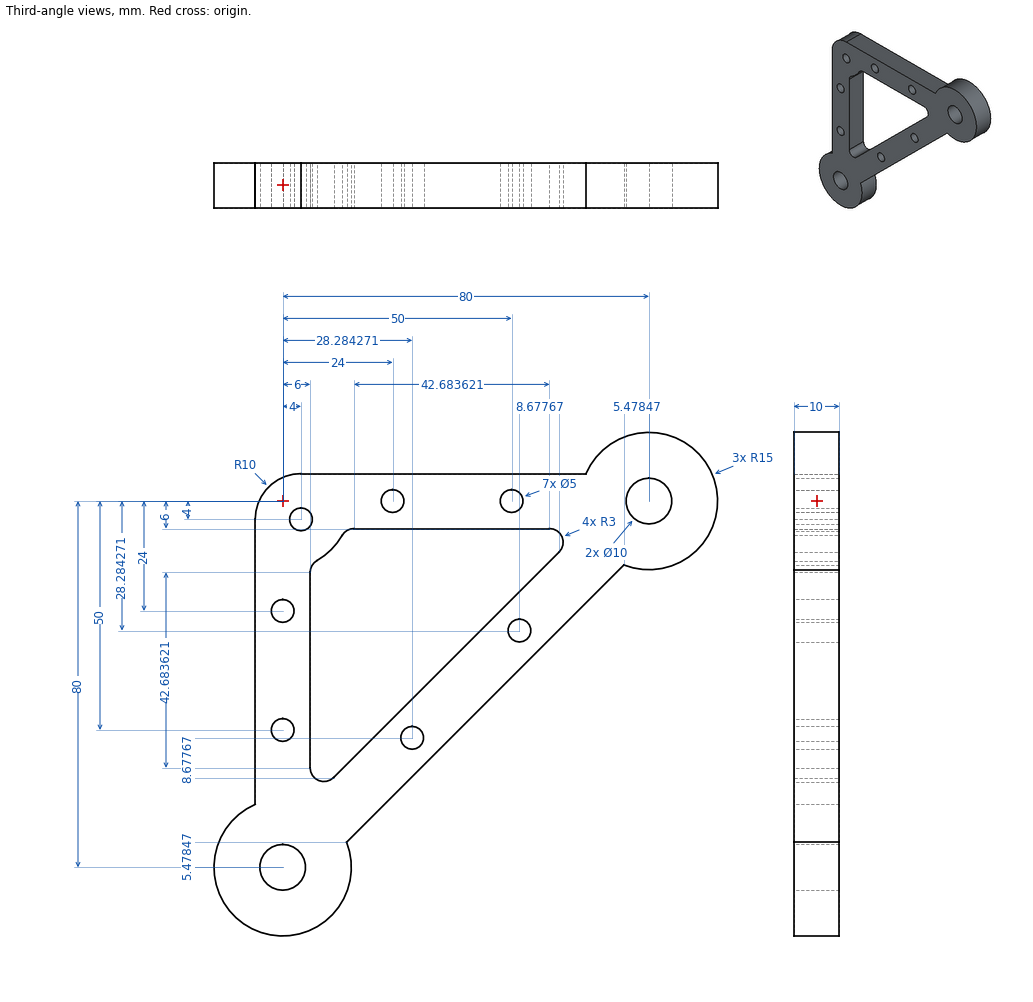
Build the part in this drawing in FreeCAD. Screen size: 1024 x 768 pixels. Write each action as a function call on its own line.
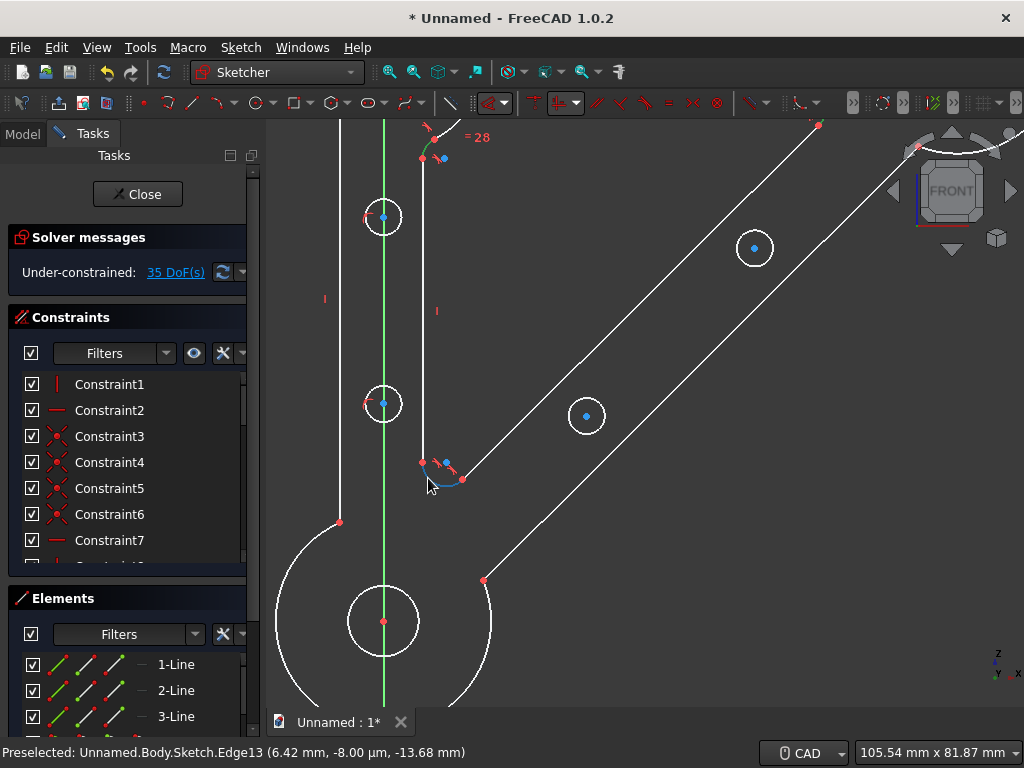
click(428, 478)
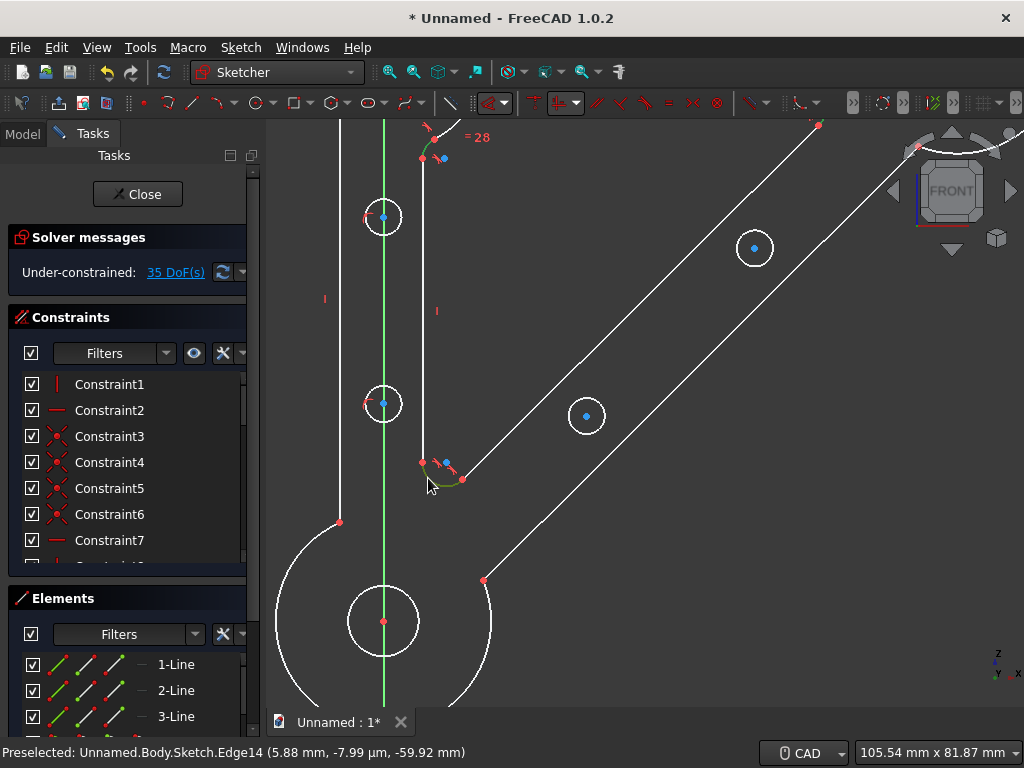
click(670, 104)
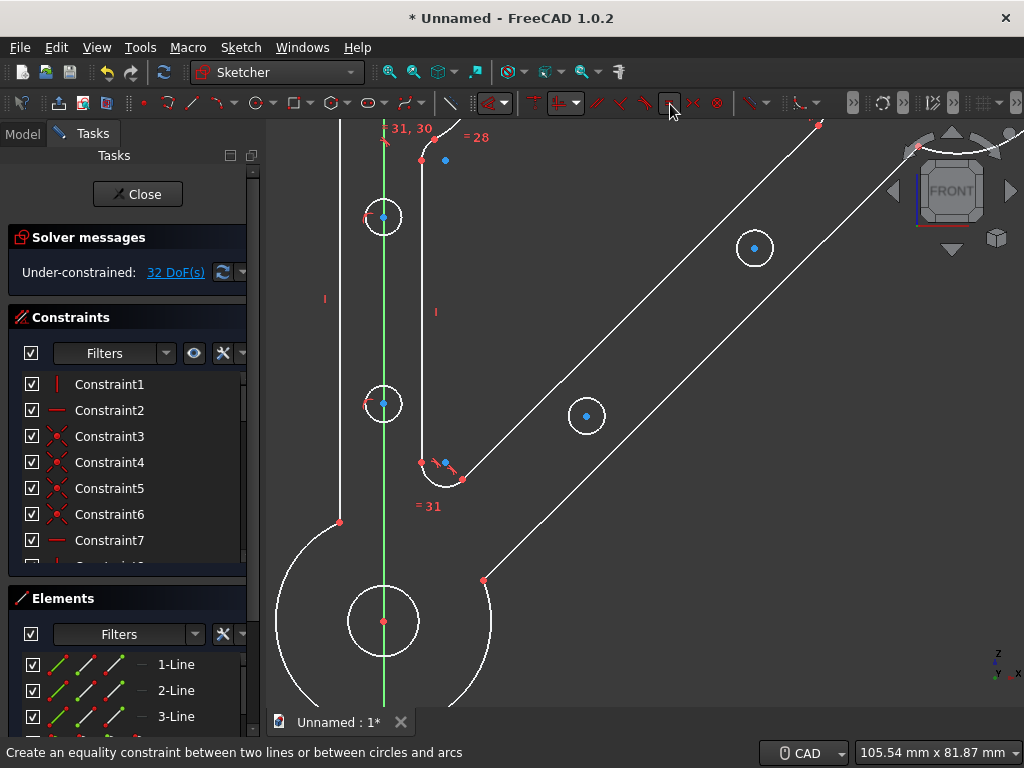
scroll(428, 478, down, 3)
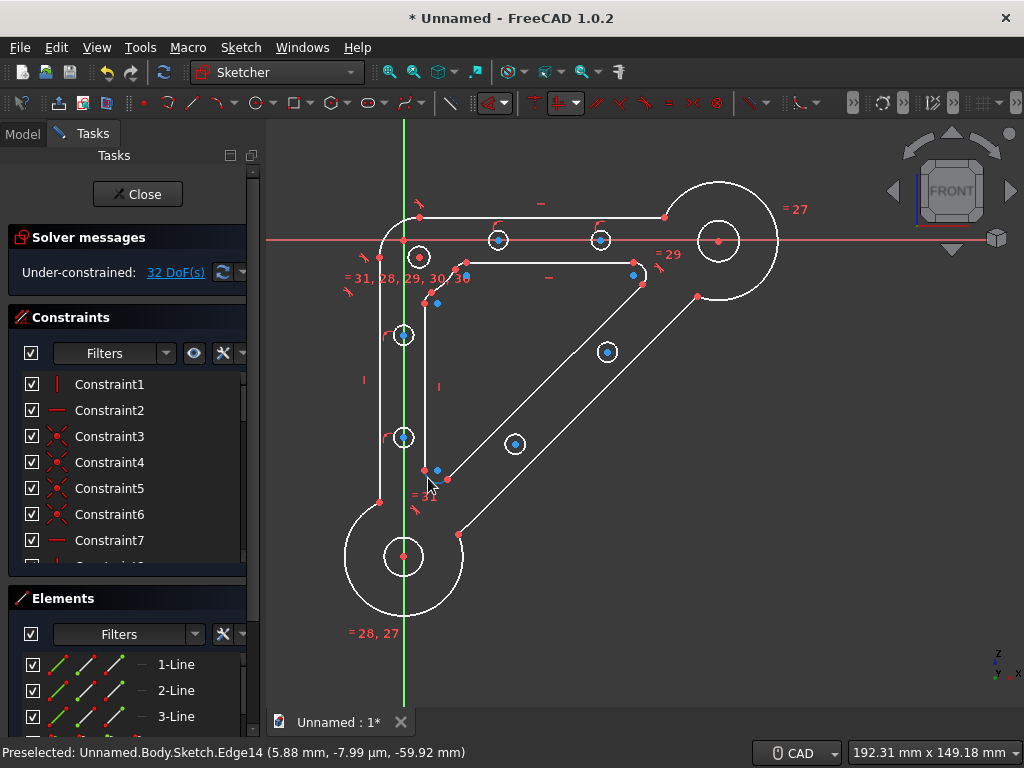
scroll(608, 233, up, 4)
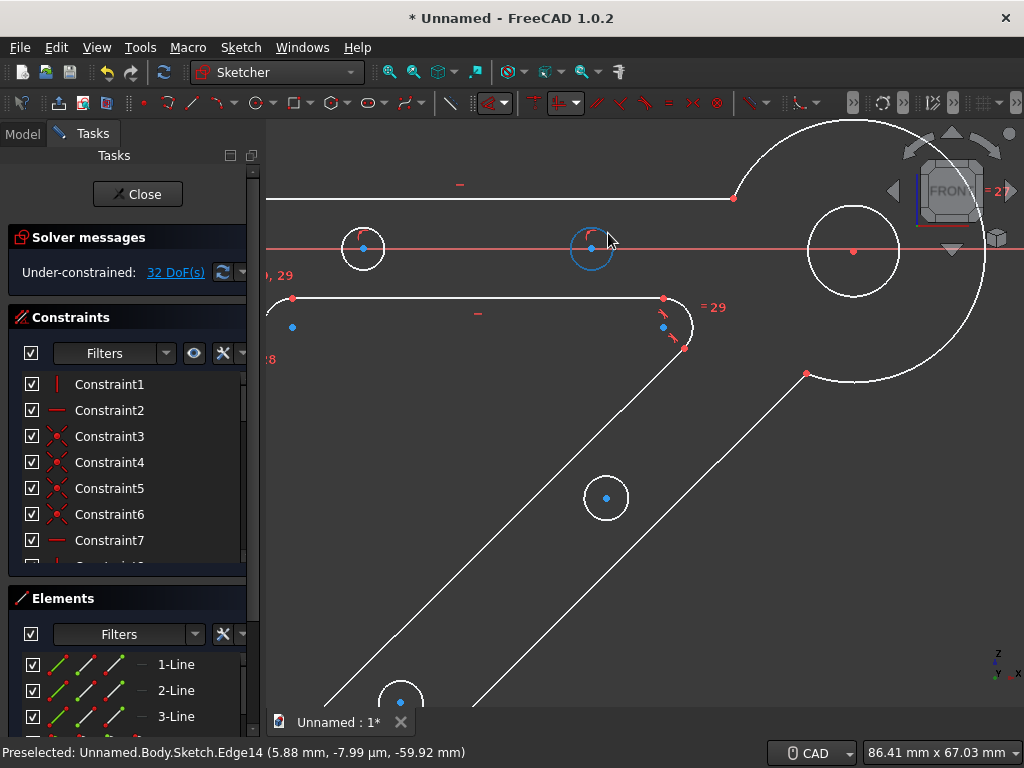
click(607, 234)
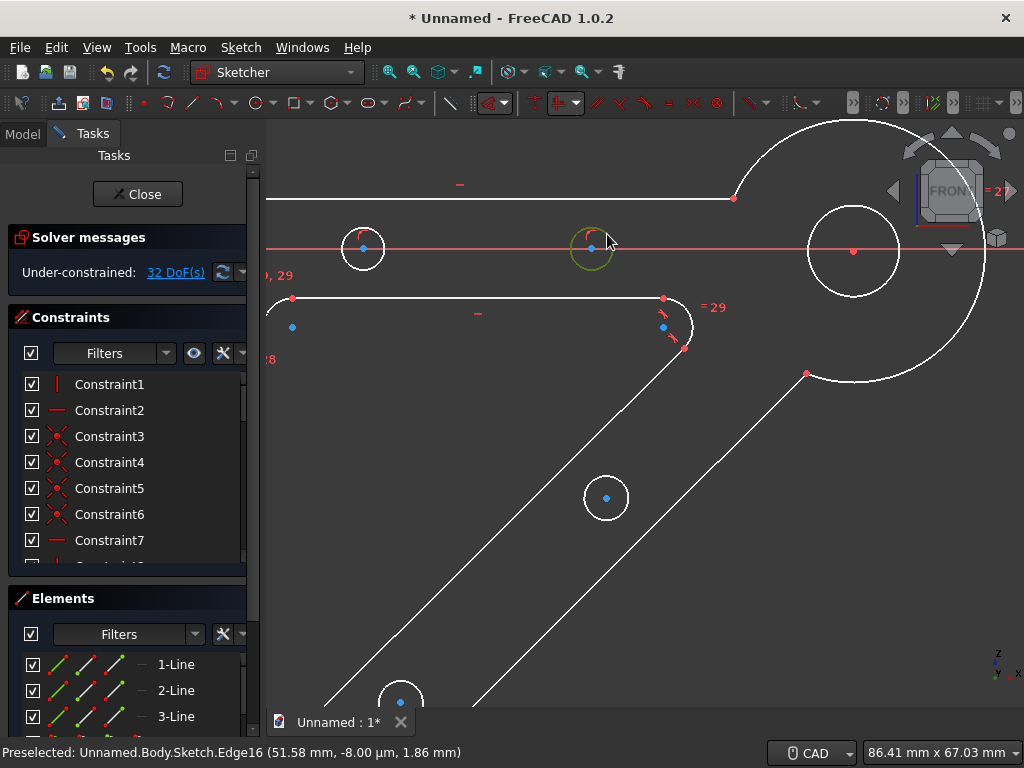
click(622, 483)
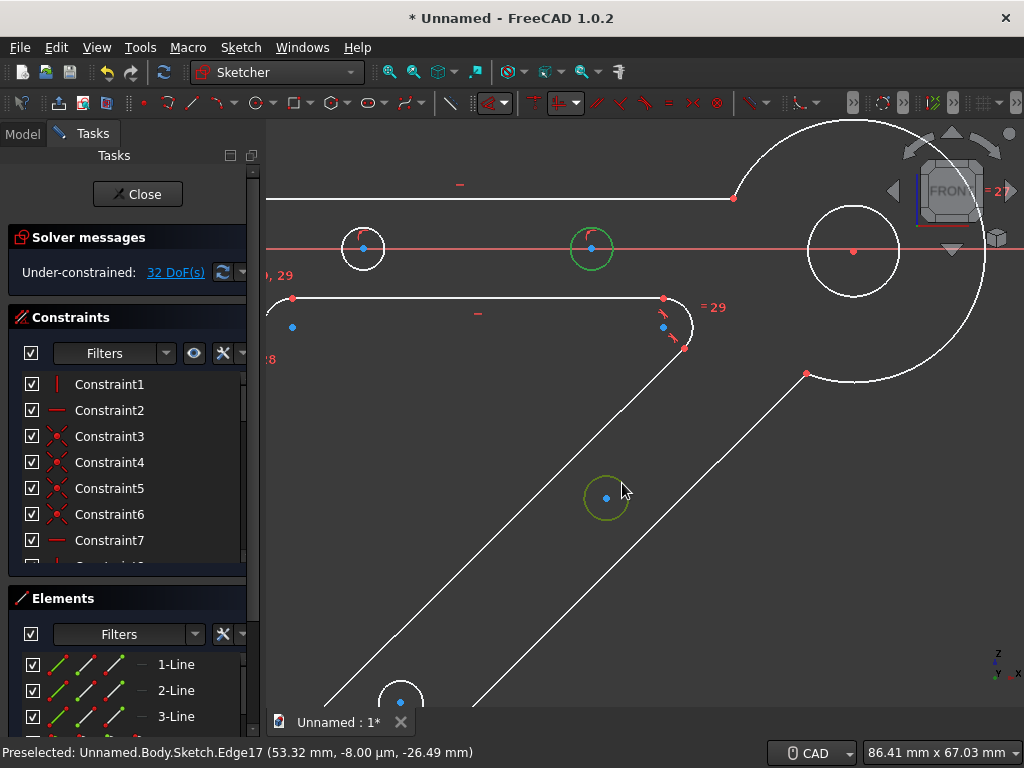
click(378, 234)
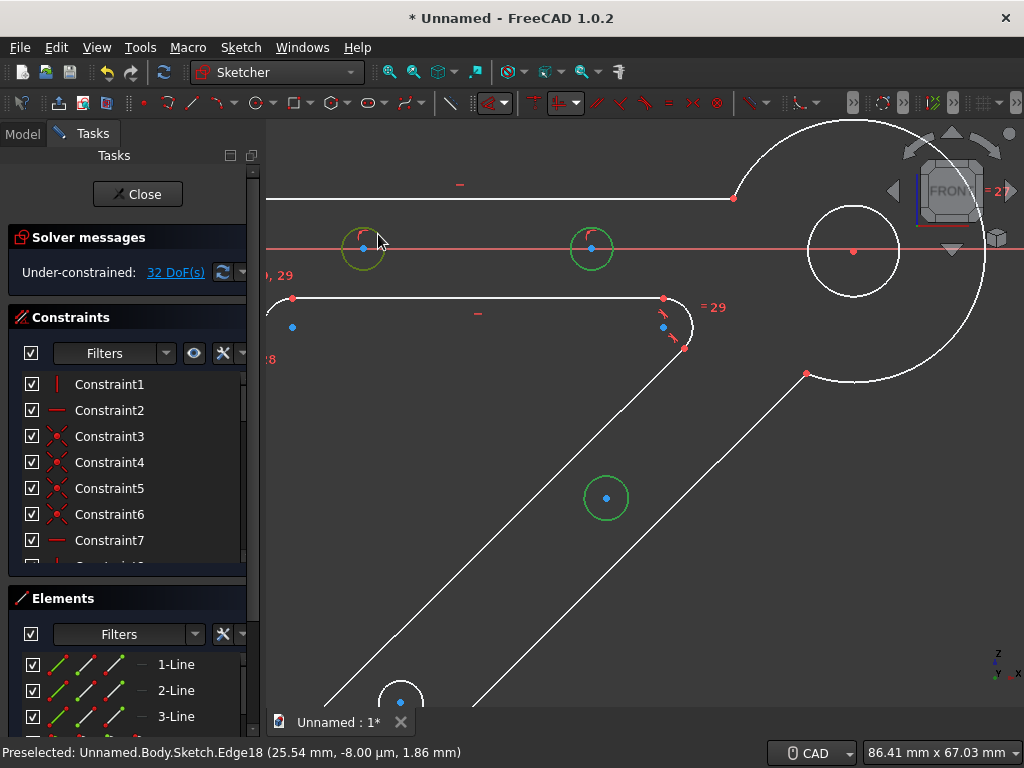
scroll(608, 233, down, 4)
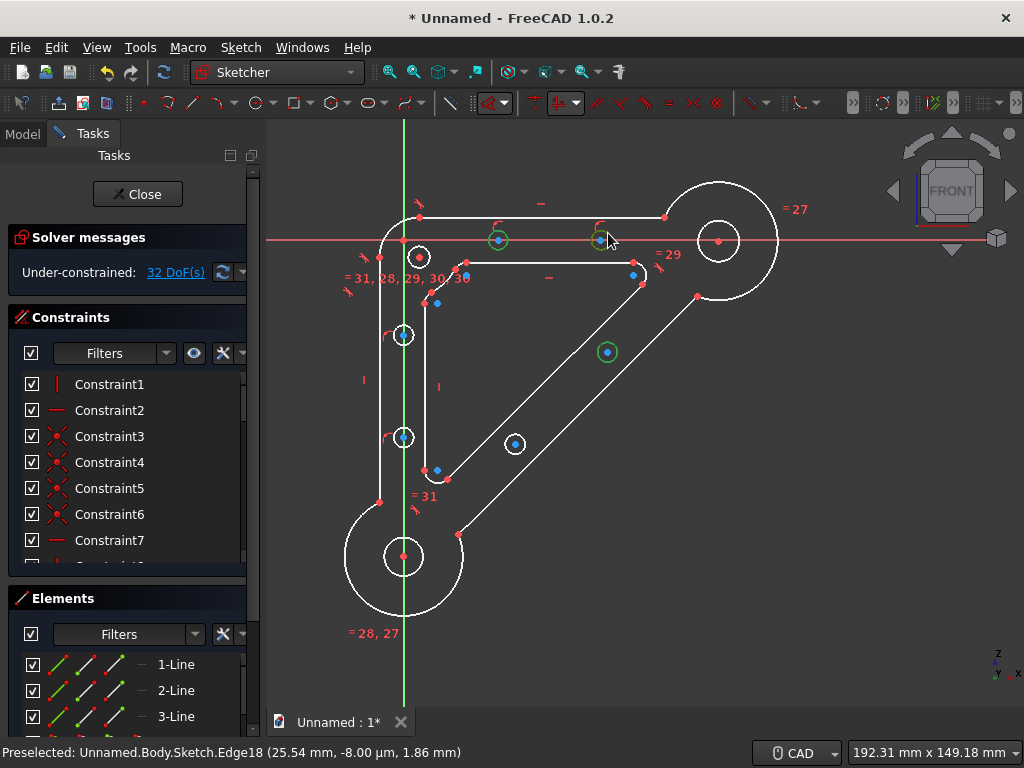
scroll(427, 250, up, 2)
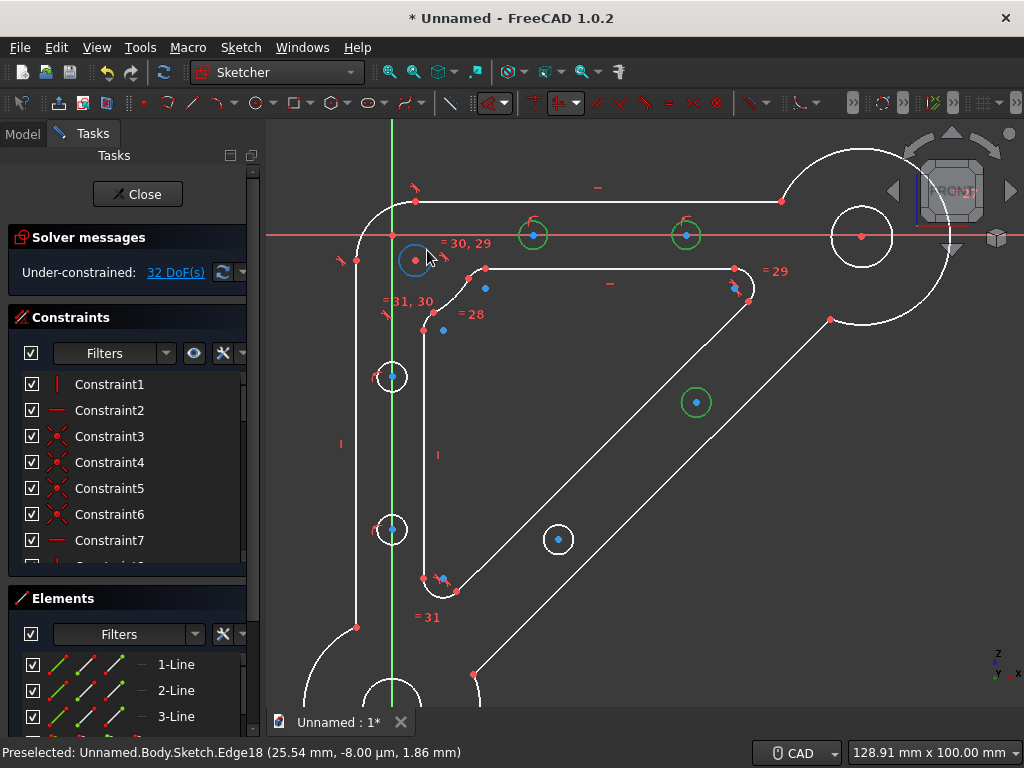
click(426, 249)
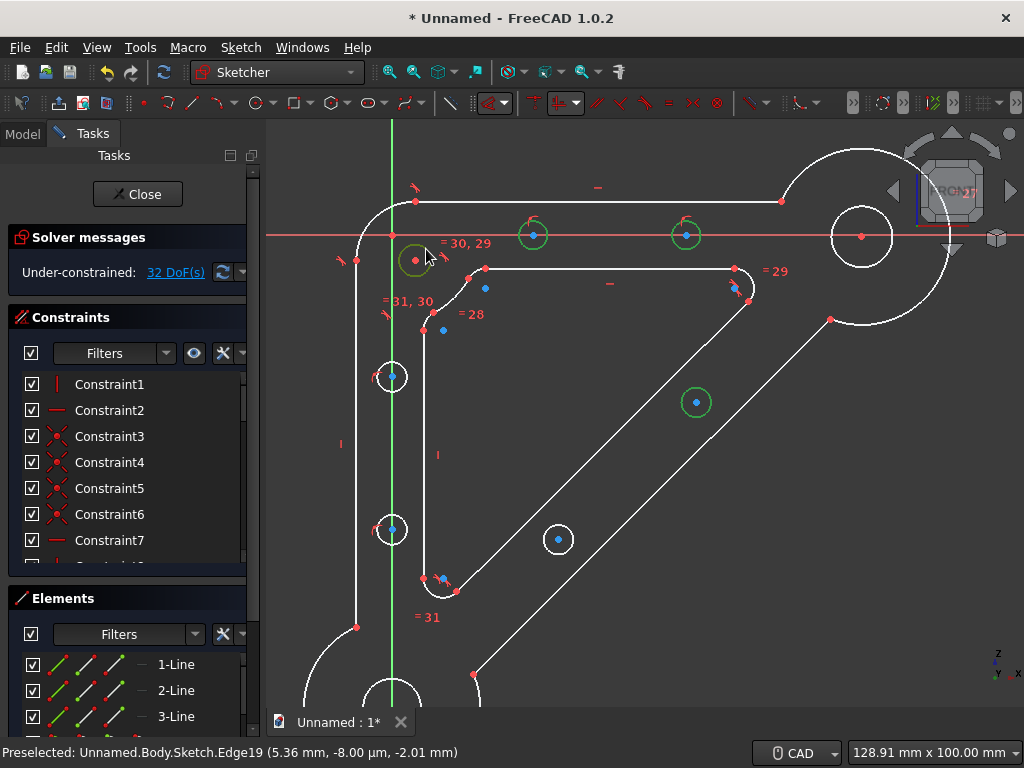
scroll(402, 366, up, 2)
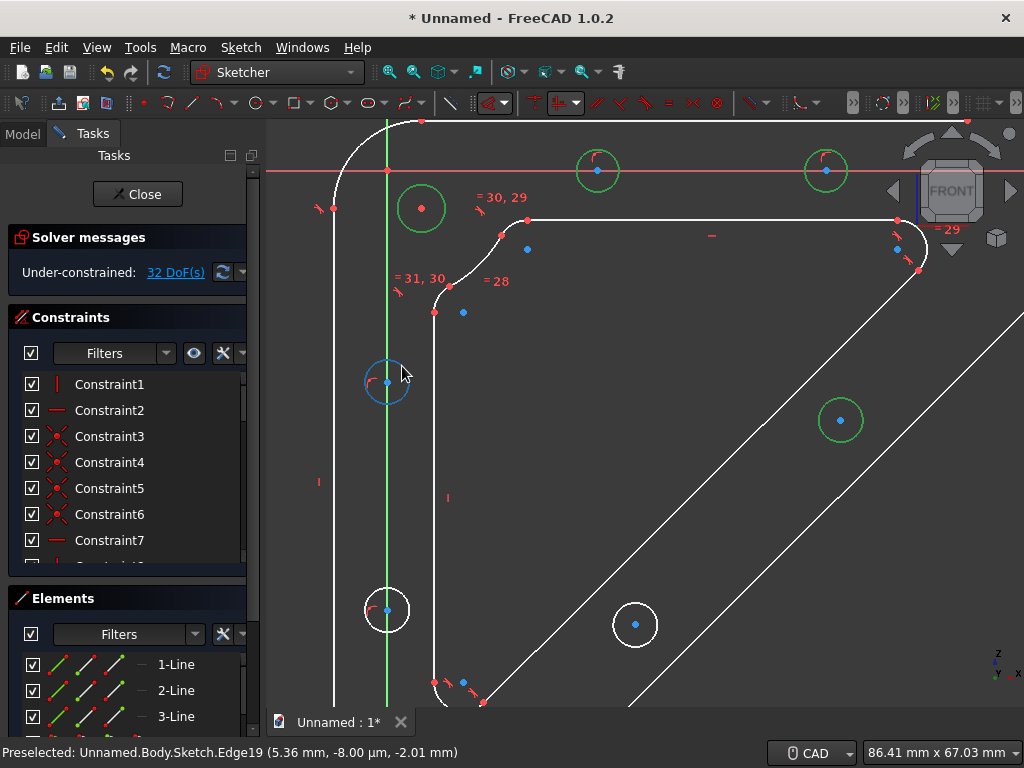
click(403, 367)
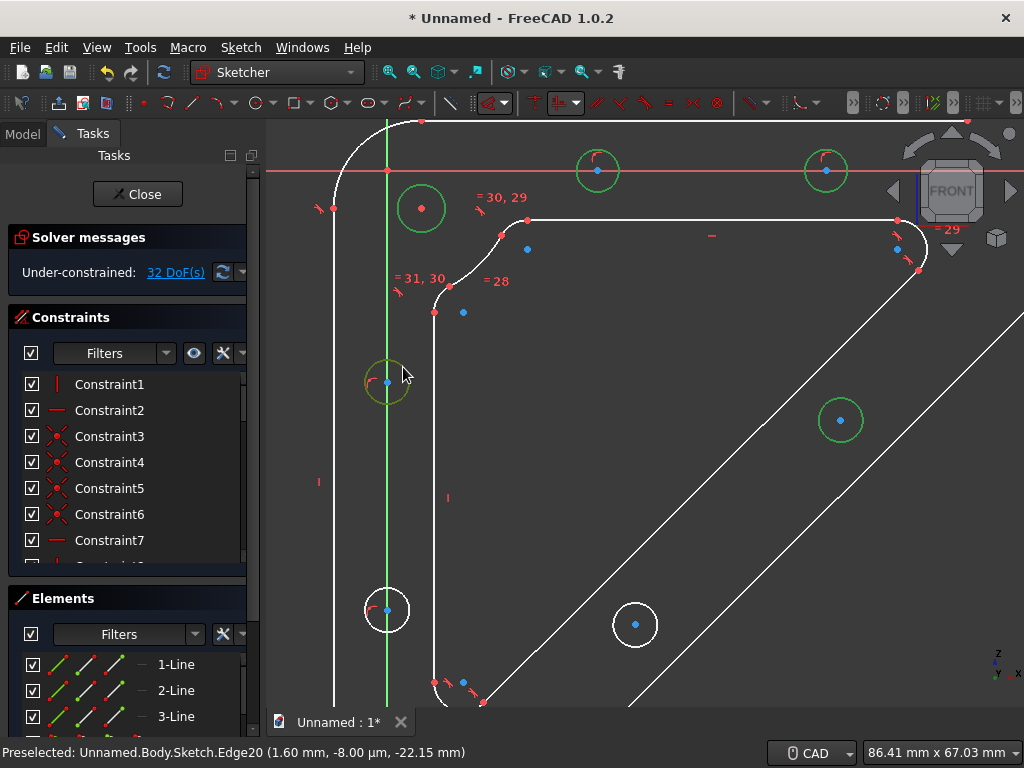
click(651, 609)